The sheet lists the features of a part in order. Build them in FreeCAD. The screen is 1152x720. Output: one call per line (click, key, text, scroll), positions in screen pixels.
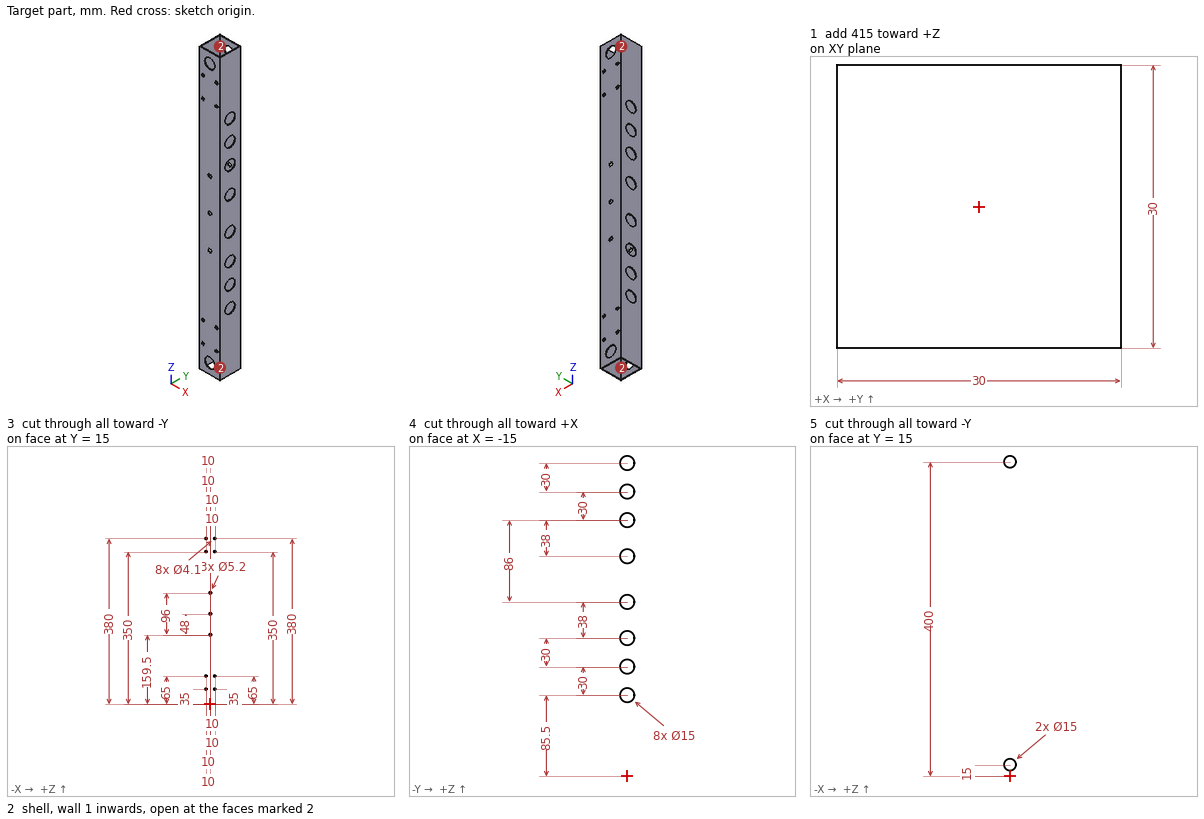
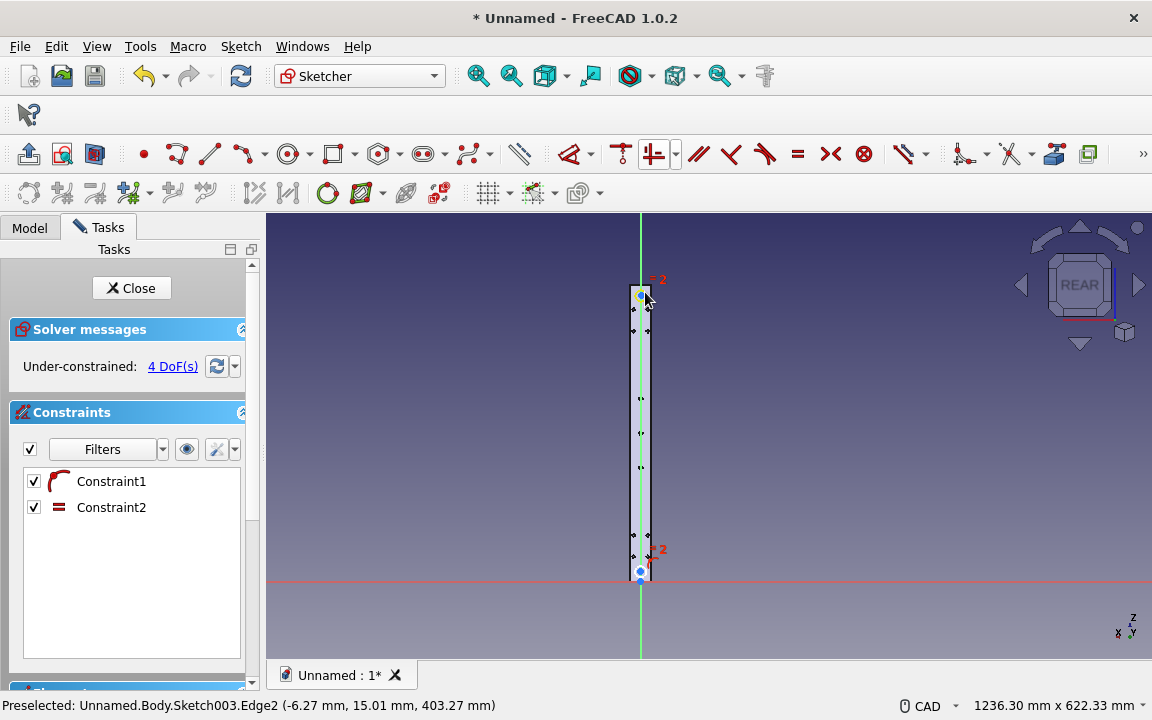
click(641, 296)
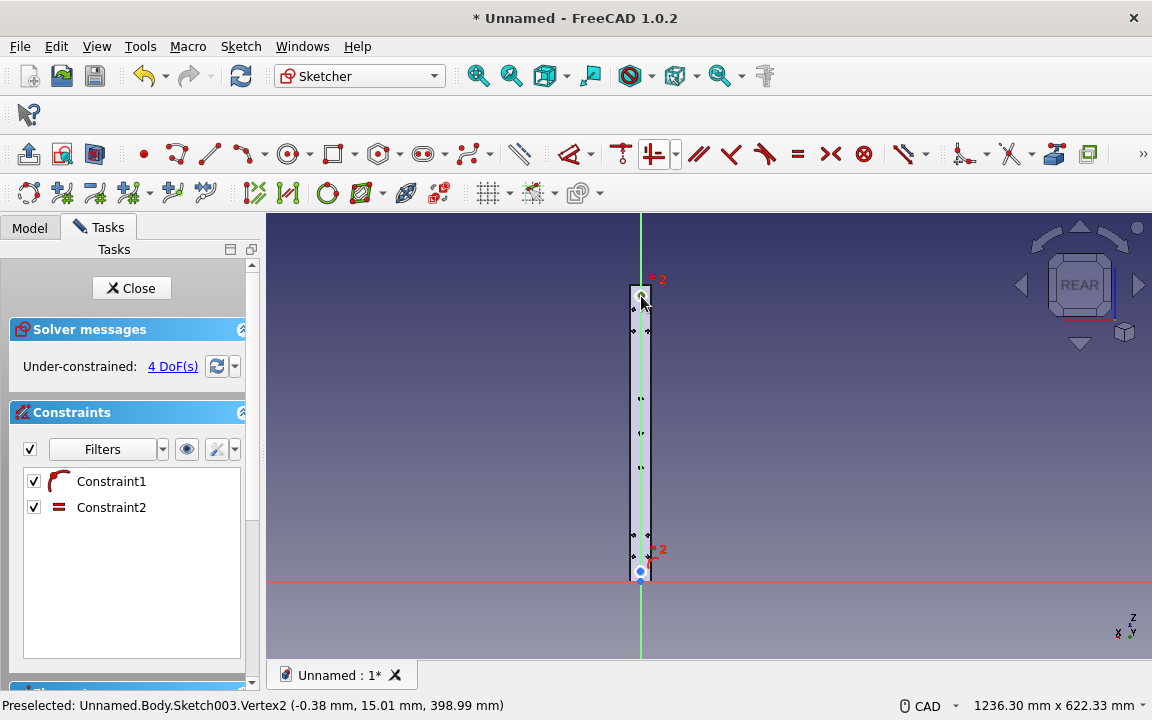
click(641, 520)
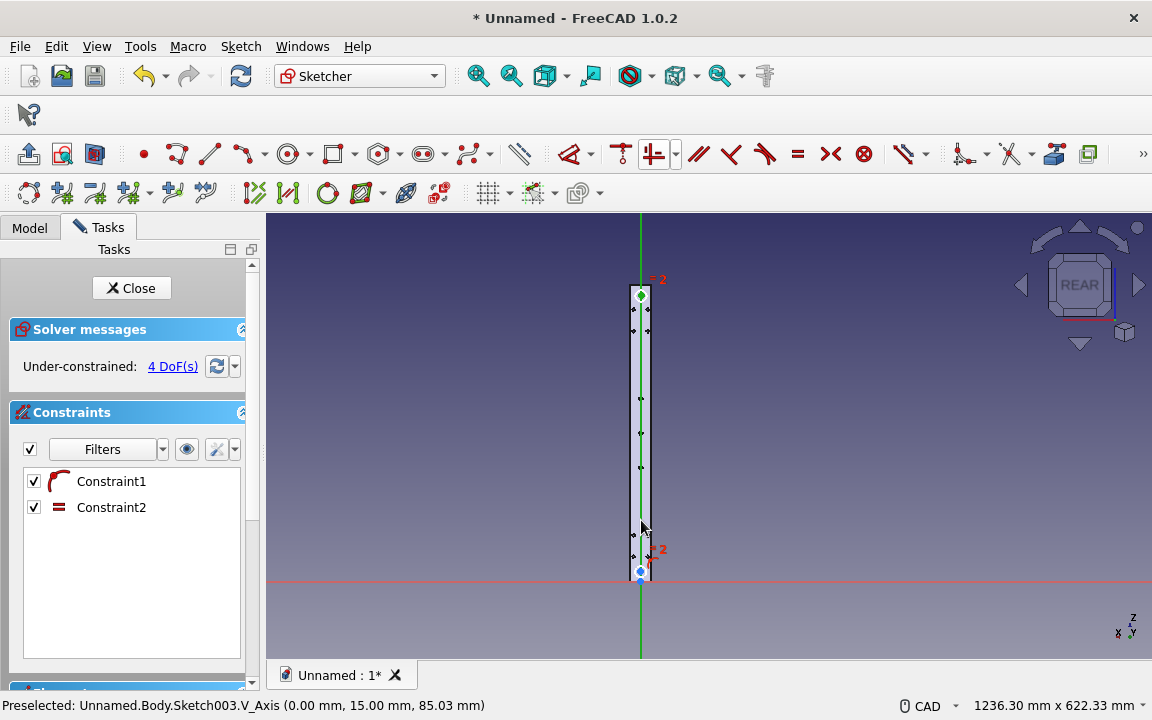
key(c)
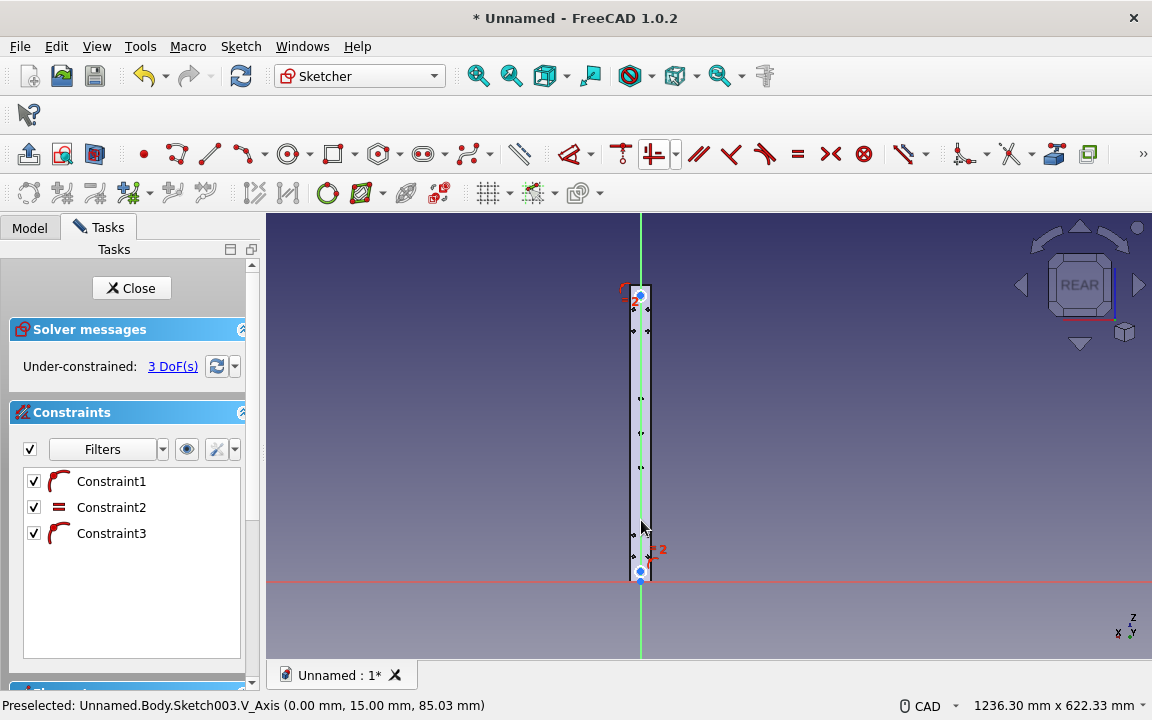
key(d)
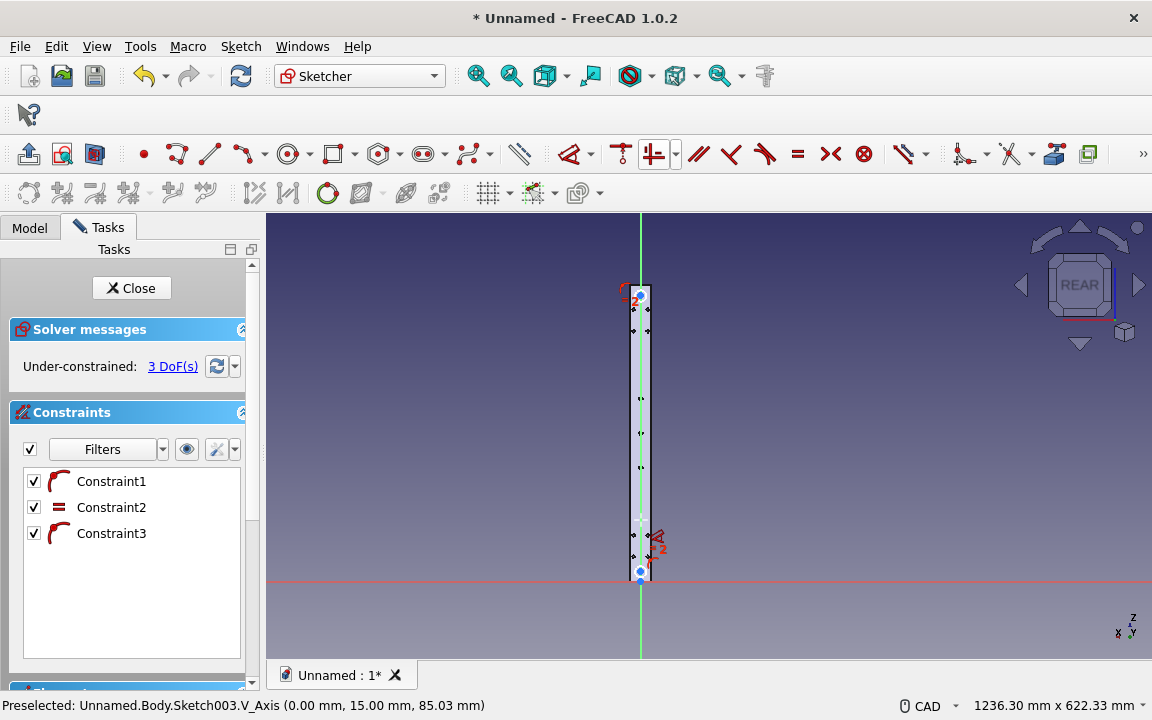
scroll(645, 568, up, 7)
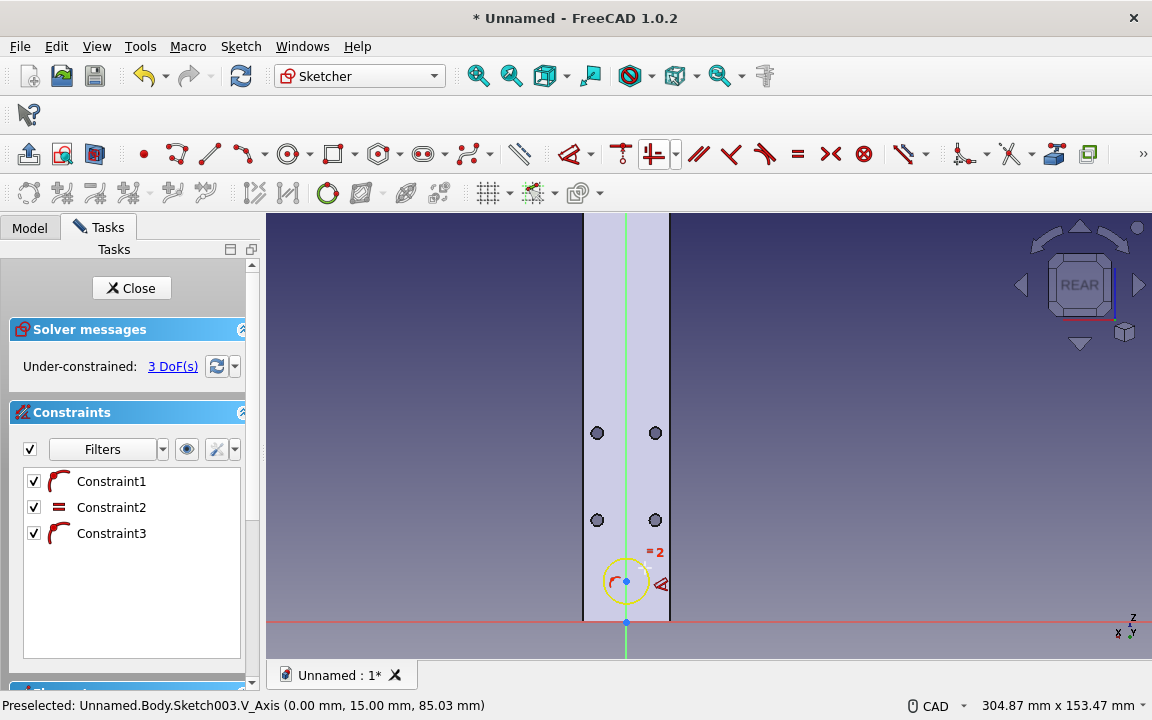
click(642, 565)
click(664, 542)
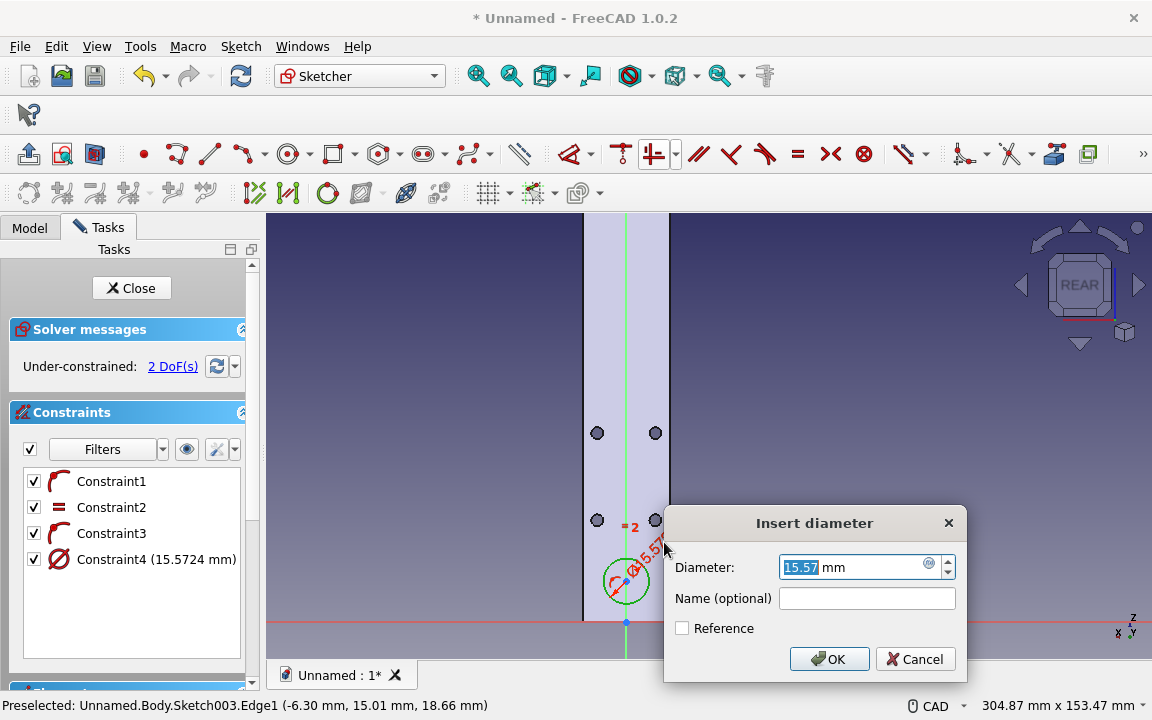
text(15)
key(Return)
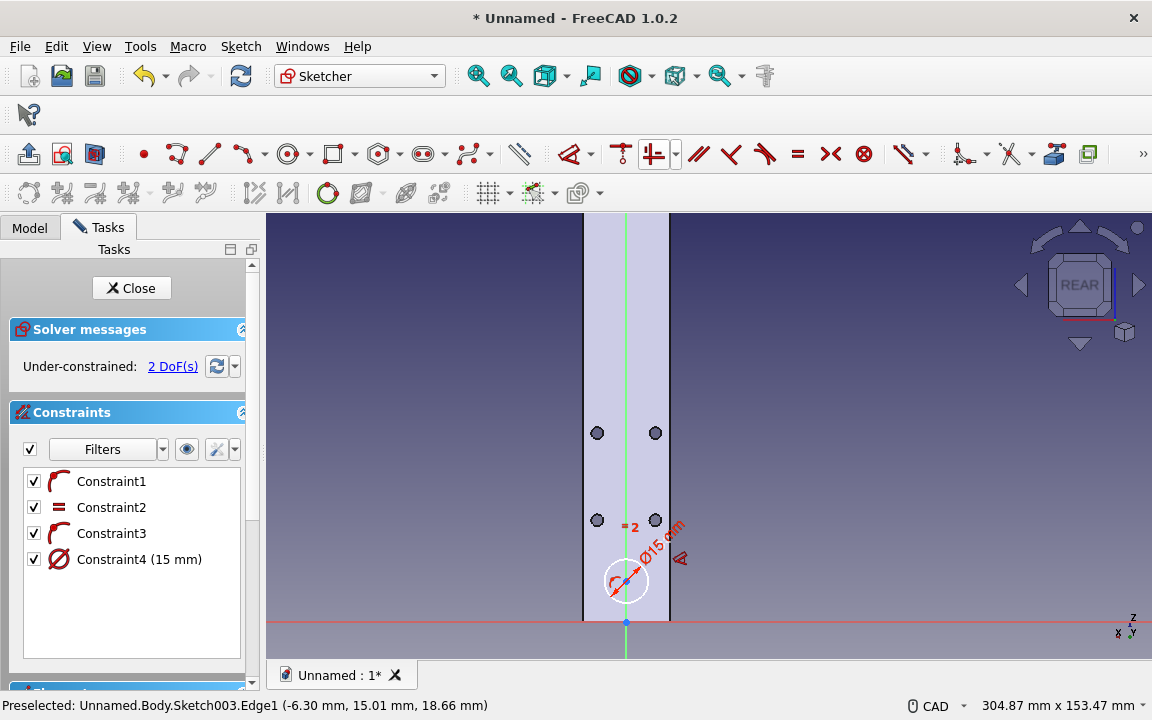
click(626, 581)
click(660, 602)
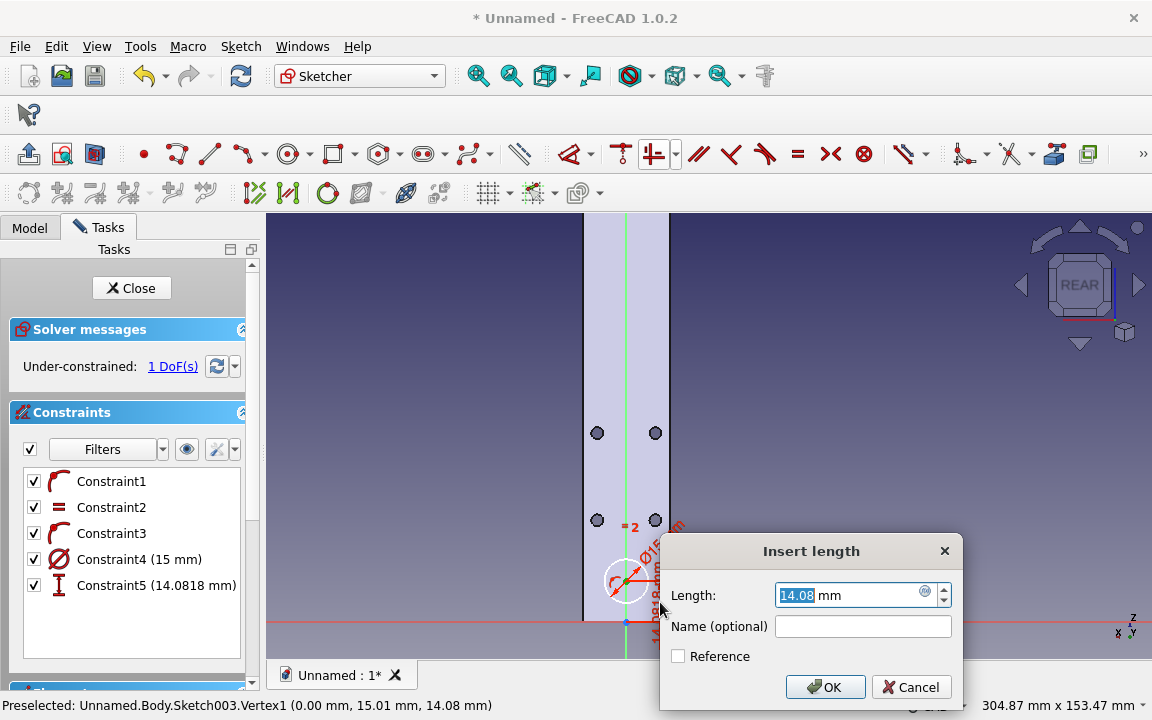
text(15)
key(Return)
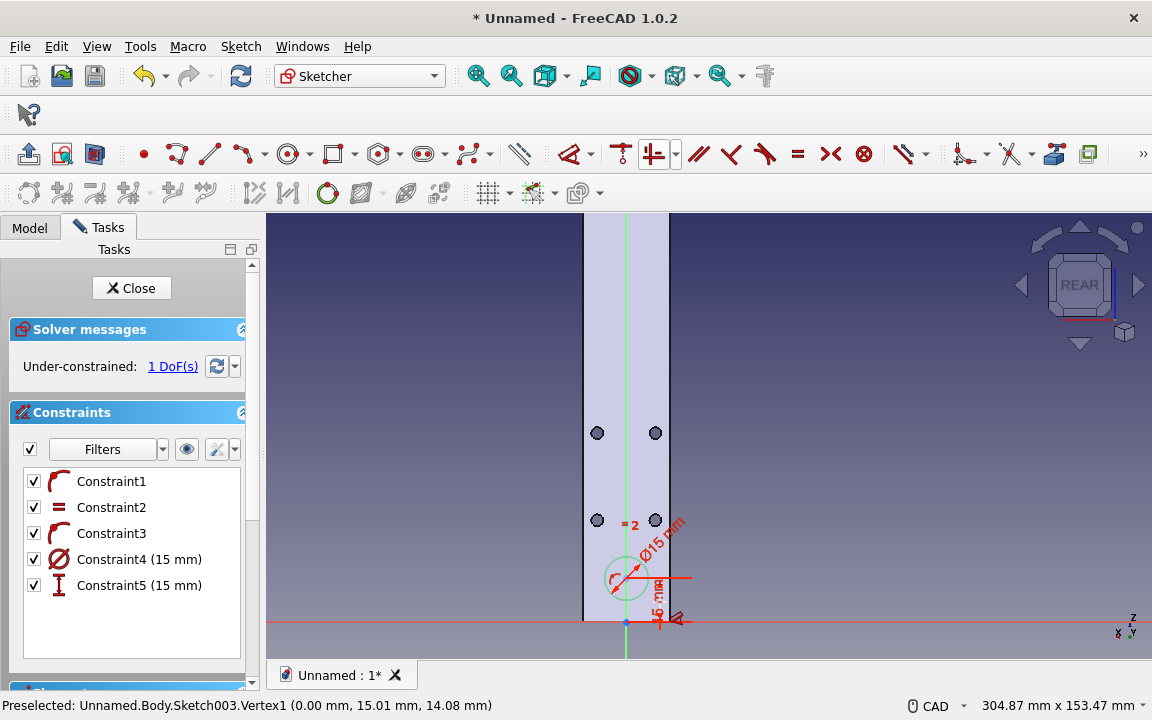
scroll(645, 569, down, 7)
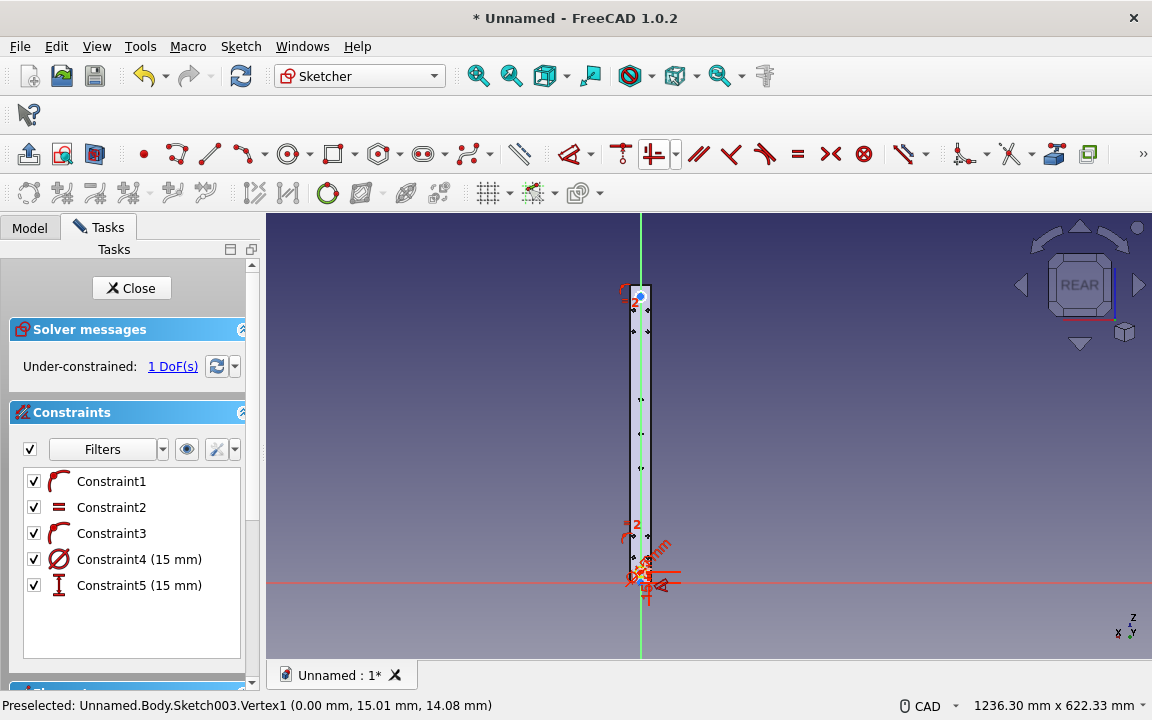
click(641, 297)
click(675, 440)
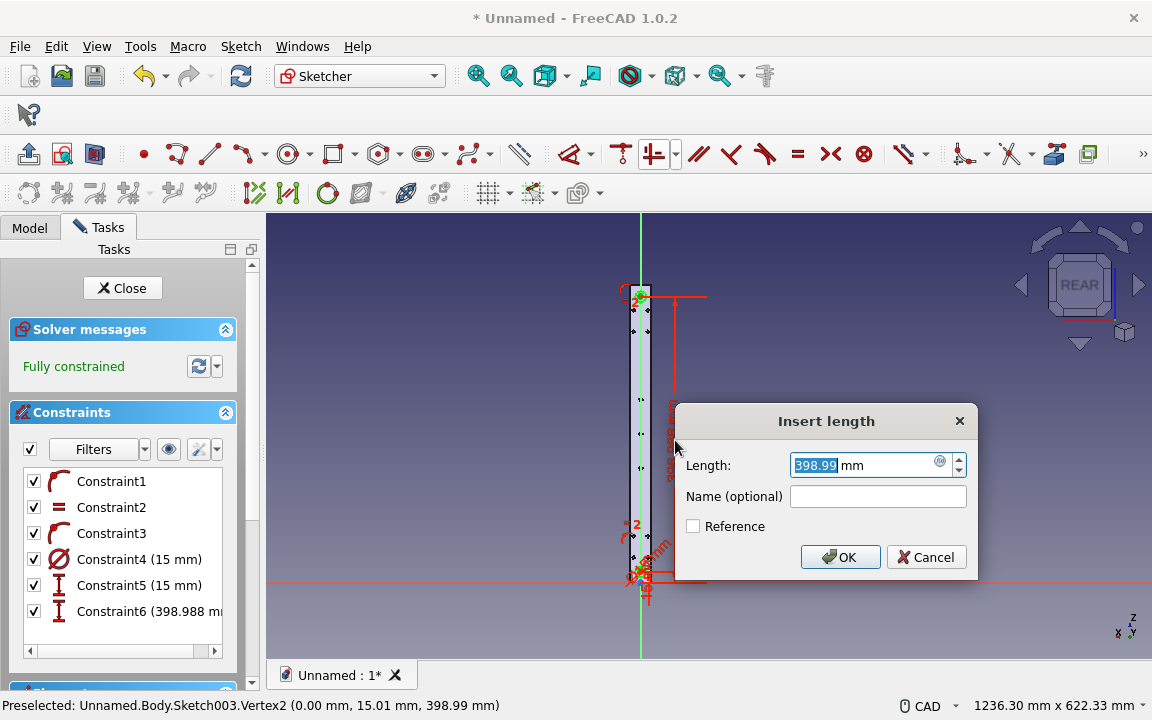
text(400)
key(Return)
key(Escape)